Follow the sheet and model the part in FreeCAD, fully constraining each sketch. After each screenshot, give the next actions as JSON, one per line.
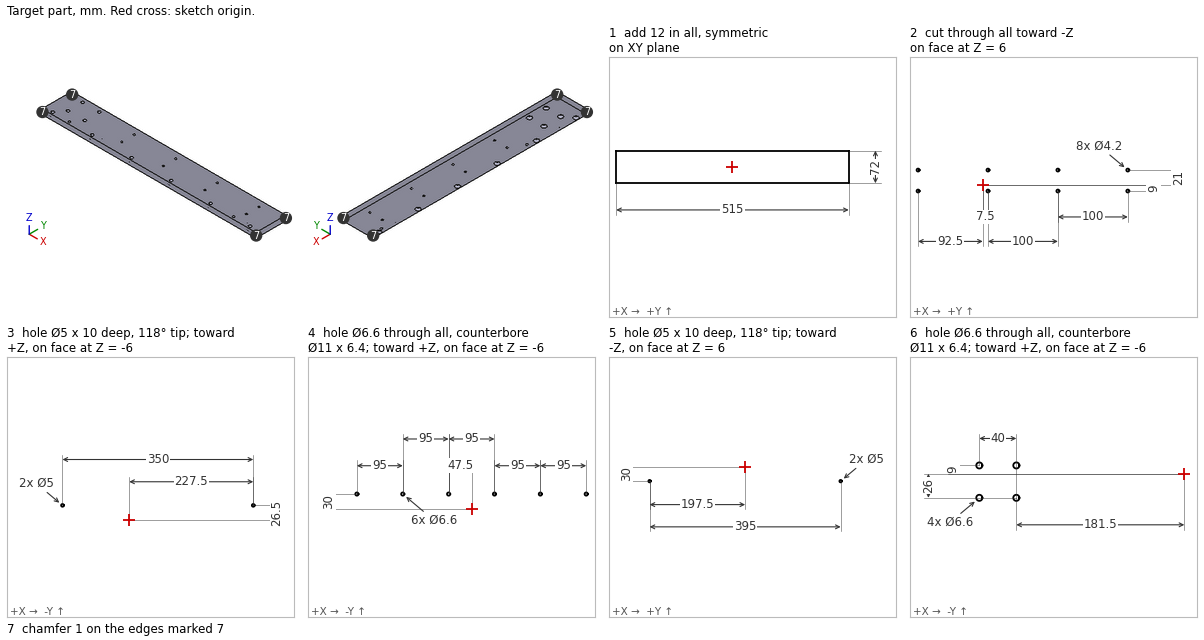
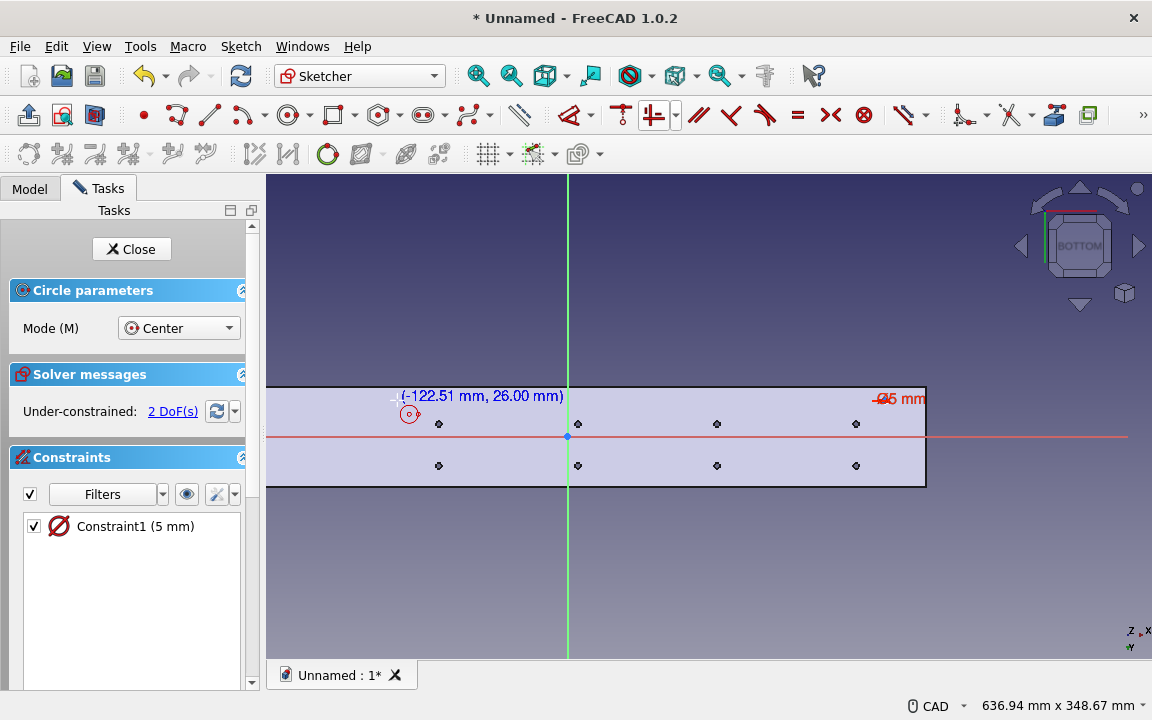
{"action": "left_click", "coordinate": [397, 400]}
{"action": "mouse_move", "coordinate": [400, 397]}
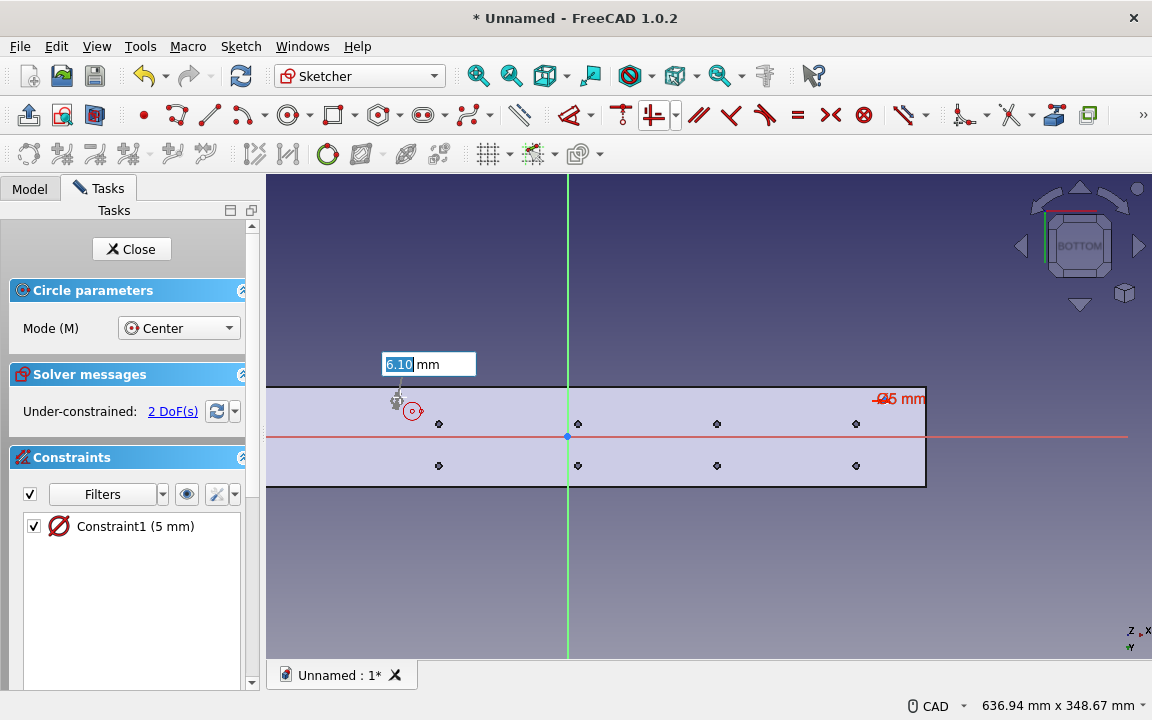
{"action": "type", "text": "5"}
{"action": "key", "text": "Return"}
{"action": "key", "text": "Escape"}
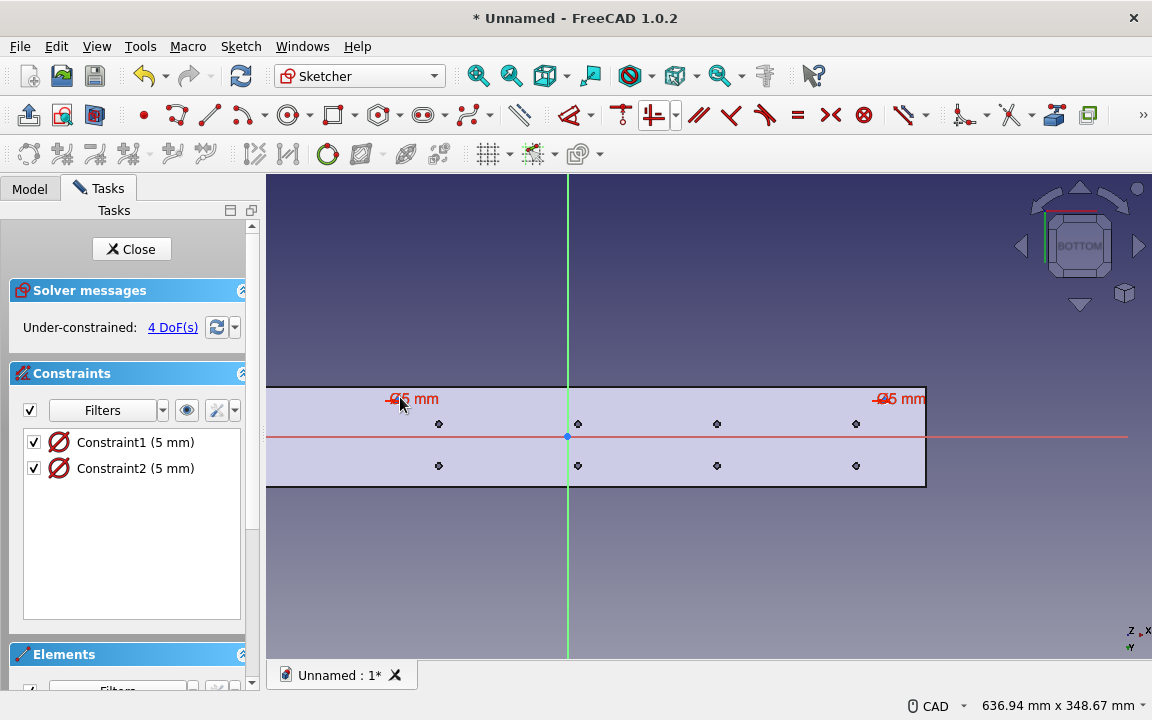
{"action": "left_click", "coordinate": [884, 401]}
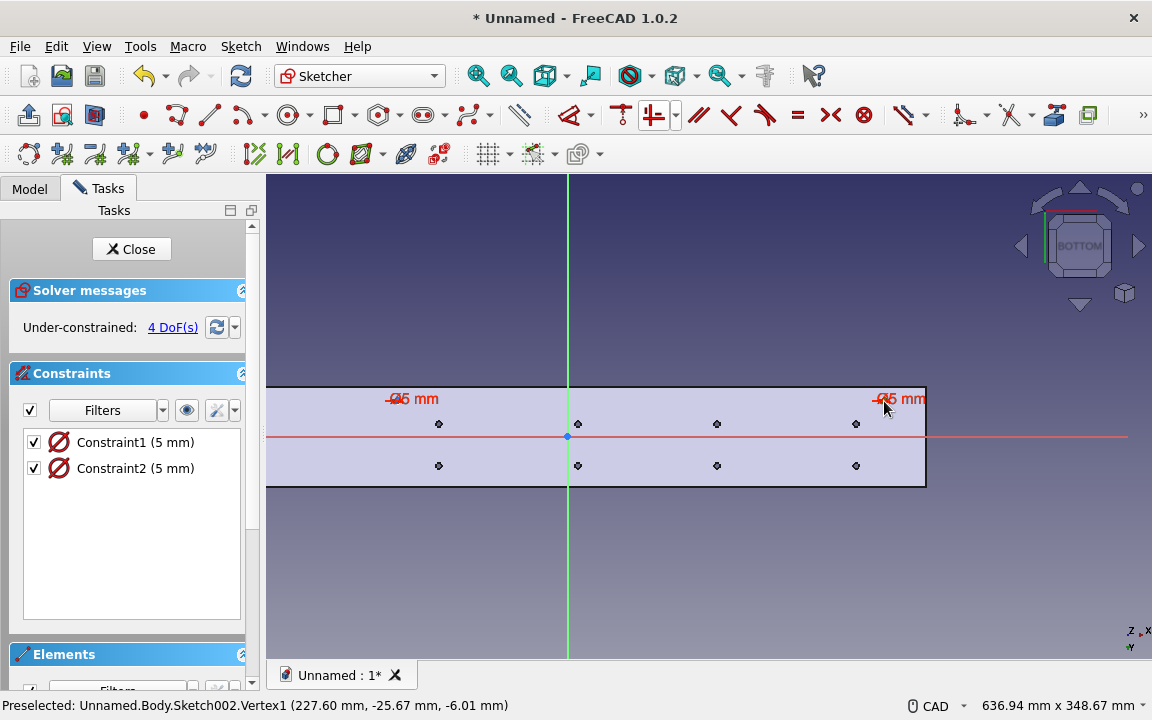
{"action": "left_click", "coordinate": [397, 401]}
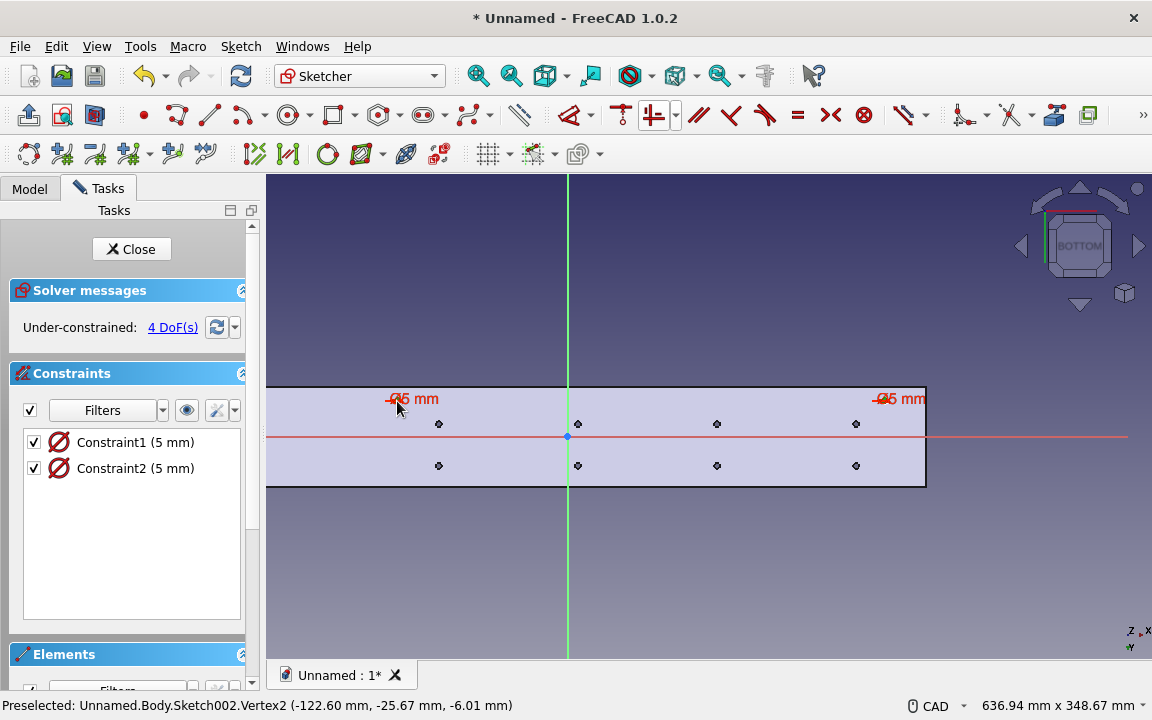
{"action": "key", "text": "h"}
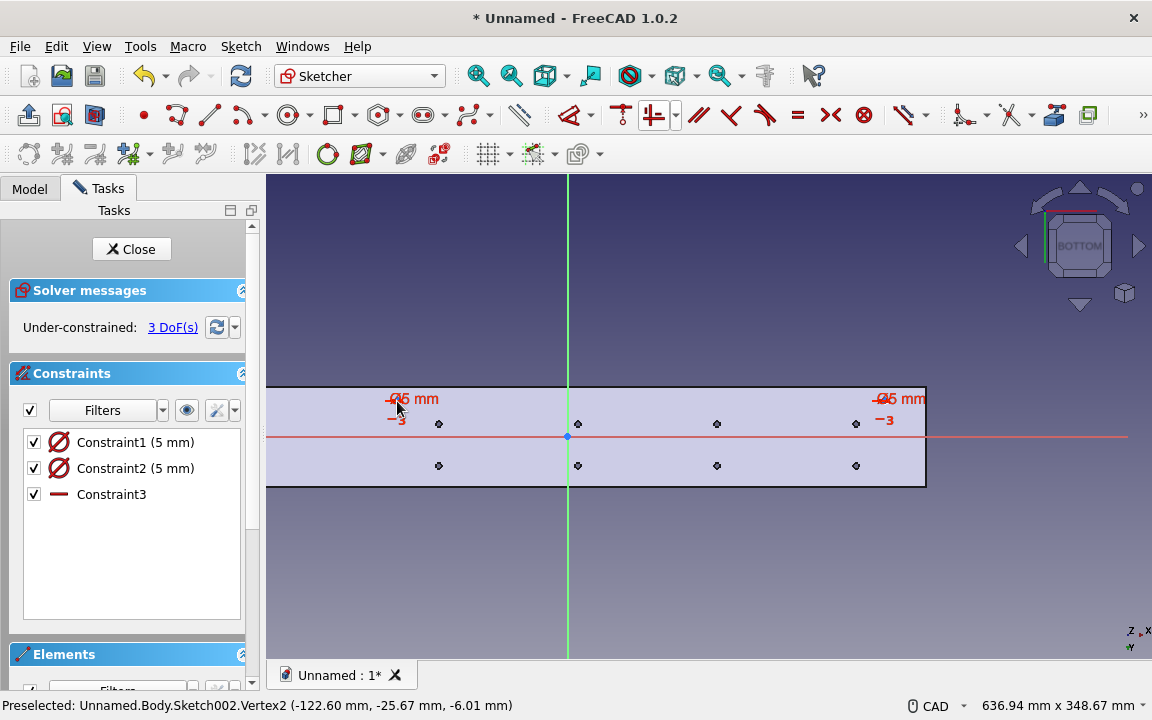
{"action": "left_click", "coordinate": [884, 401]}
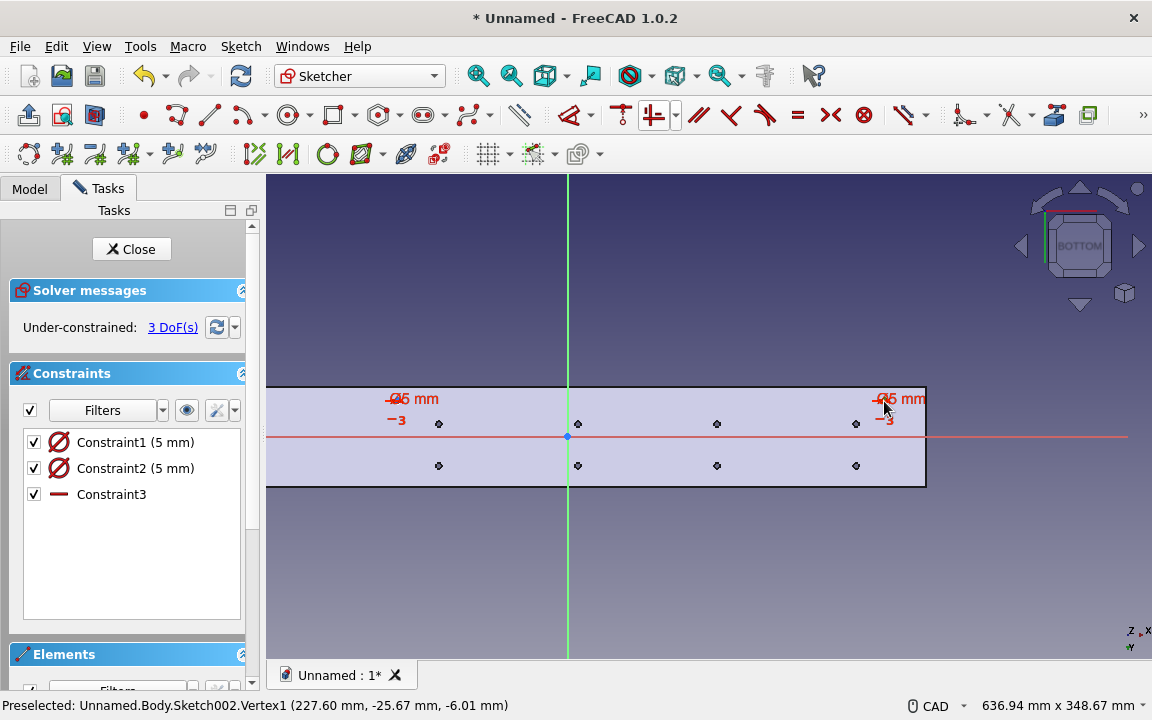
{"action": "left_click", "coordinate": [590, 116]}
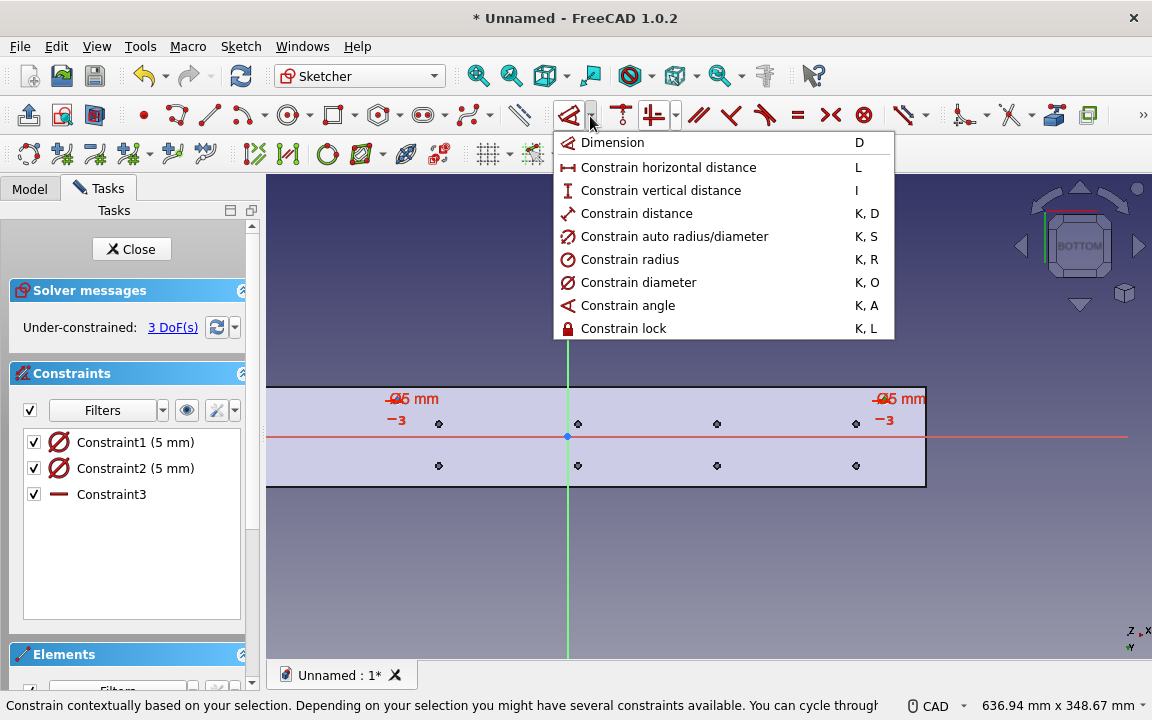
{"action": "left_click", "coordinate": [724, 190]}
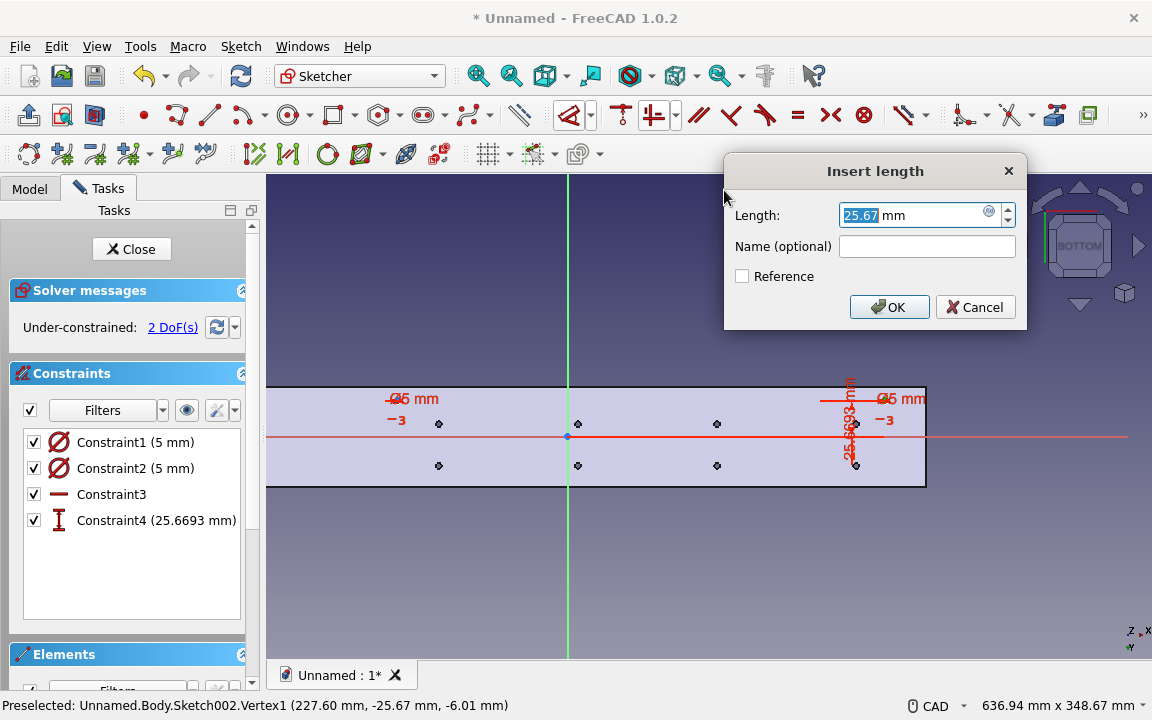
{"action": "type", "text": "26.5"}
{"action": "key", "text": "Return"}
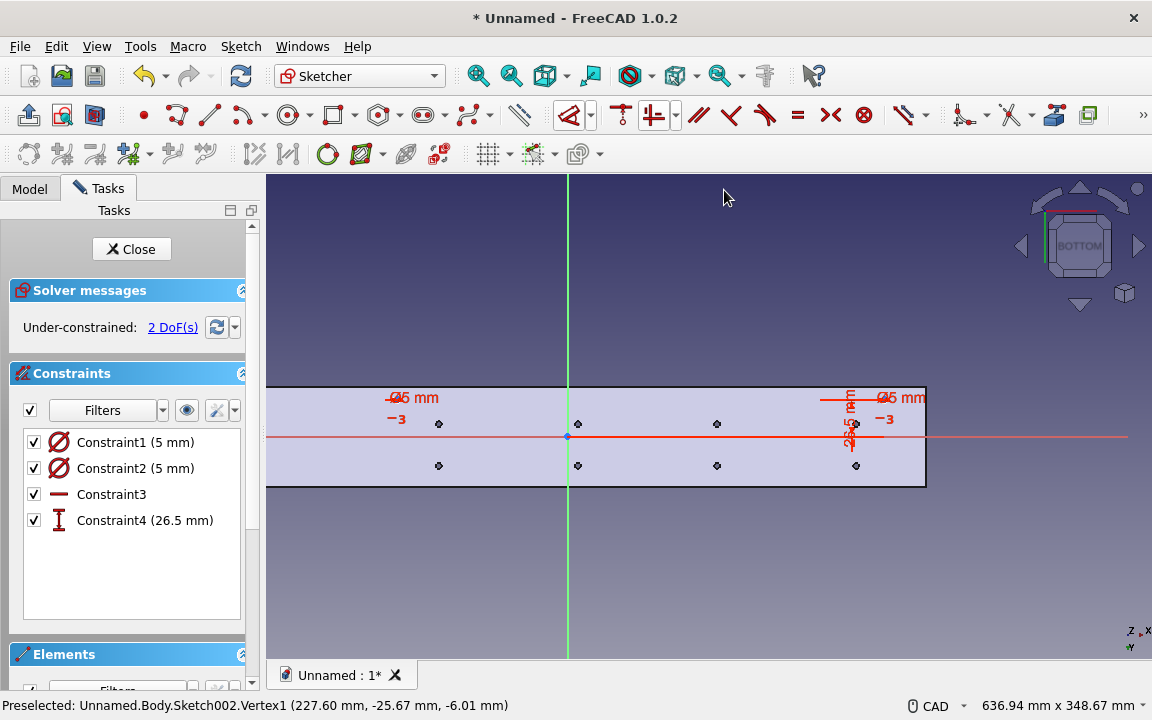
{"action": "left_click", "coordinate": [884, 400]}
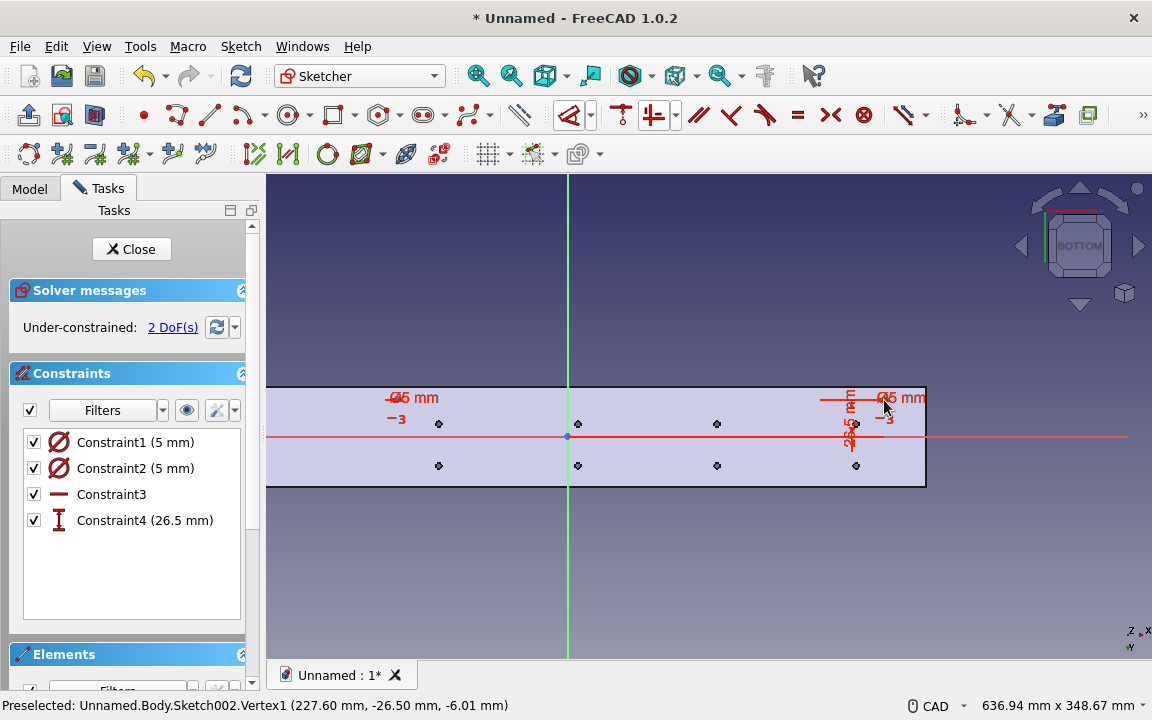
{"action": "left_click", "coordinate": [397, 400]}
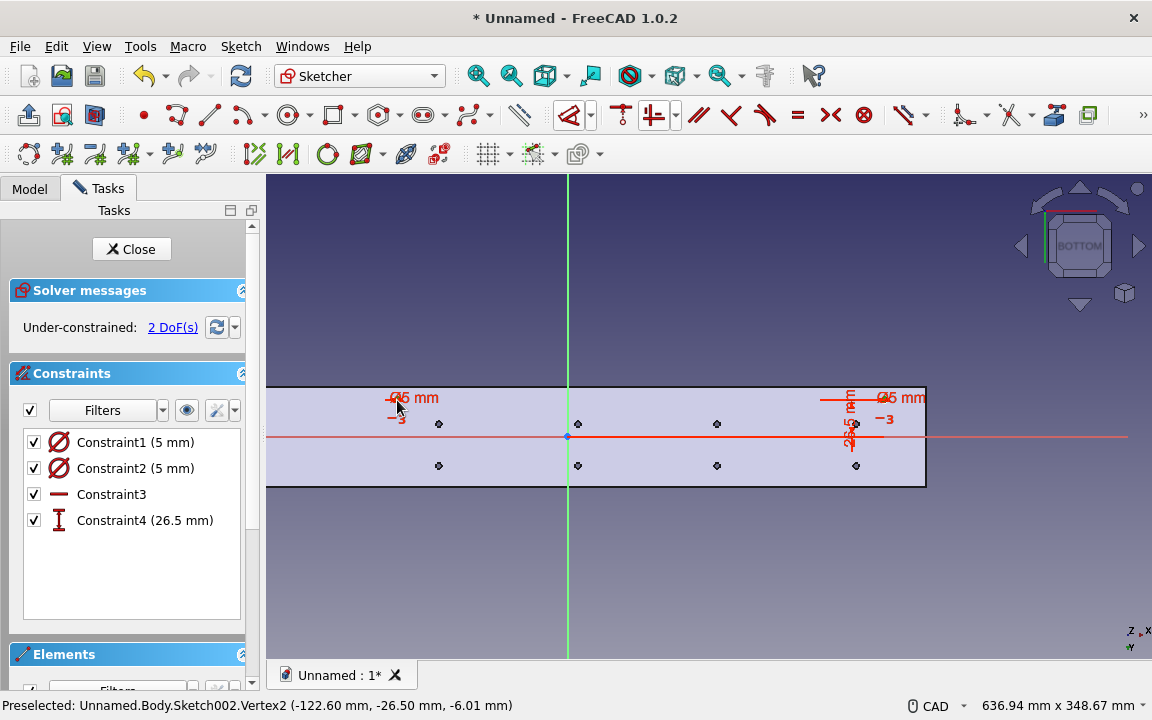
{"action": "key", "text": "l"}